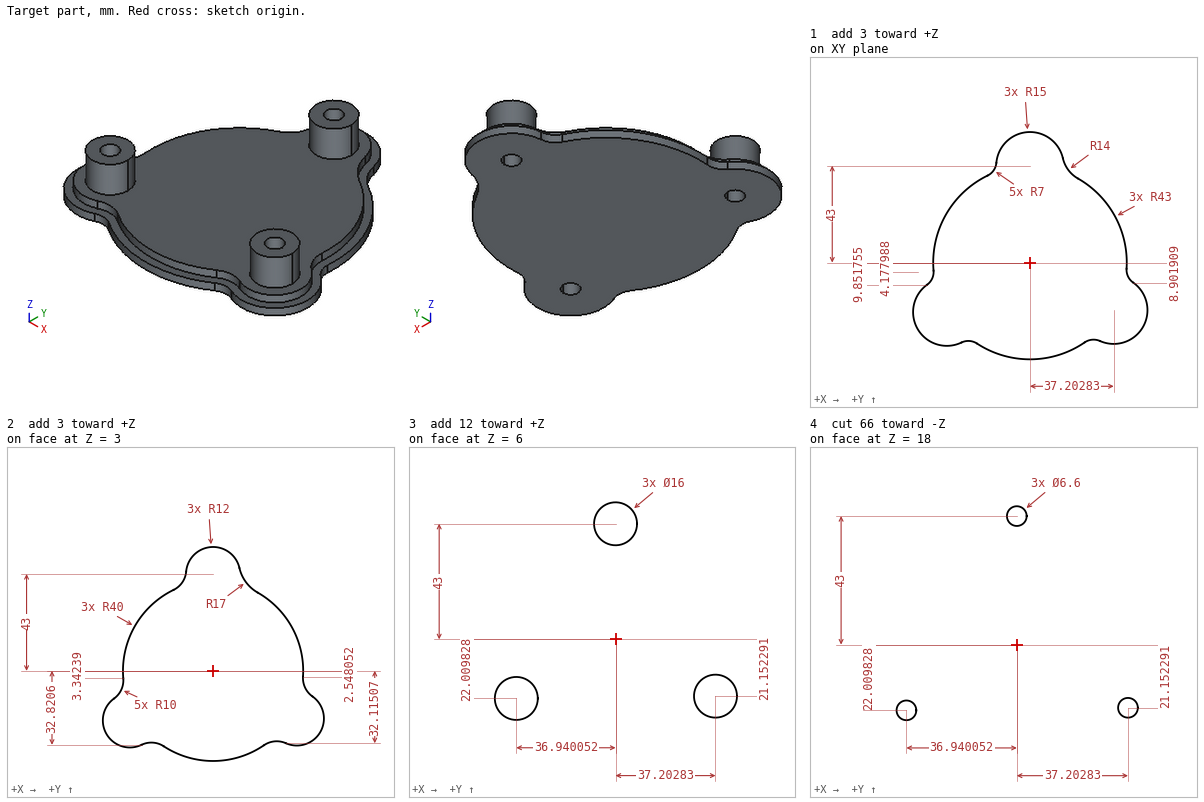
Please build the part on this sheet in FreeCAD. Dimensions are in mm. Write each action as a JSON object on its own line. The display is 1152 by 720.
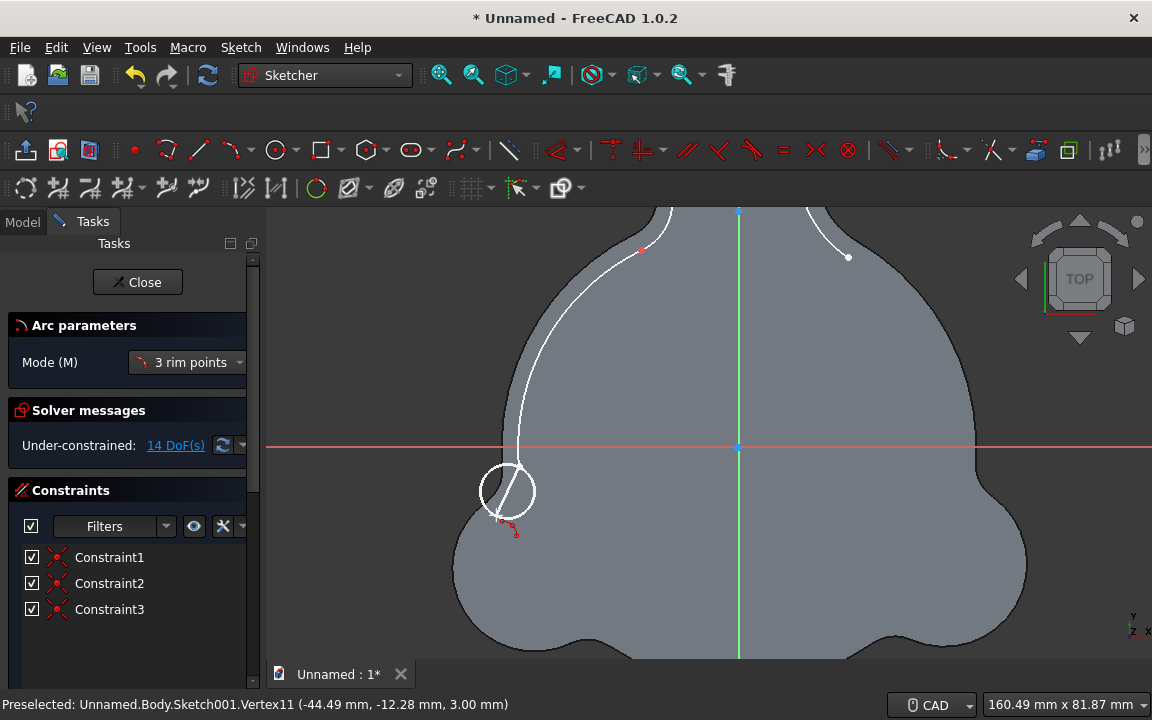
{"action": "scroll", "coordinate": [514, 493], "scroll_direction": "up", "scroll_amount": 4}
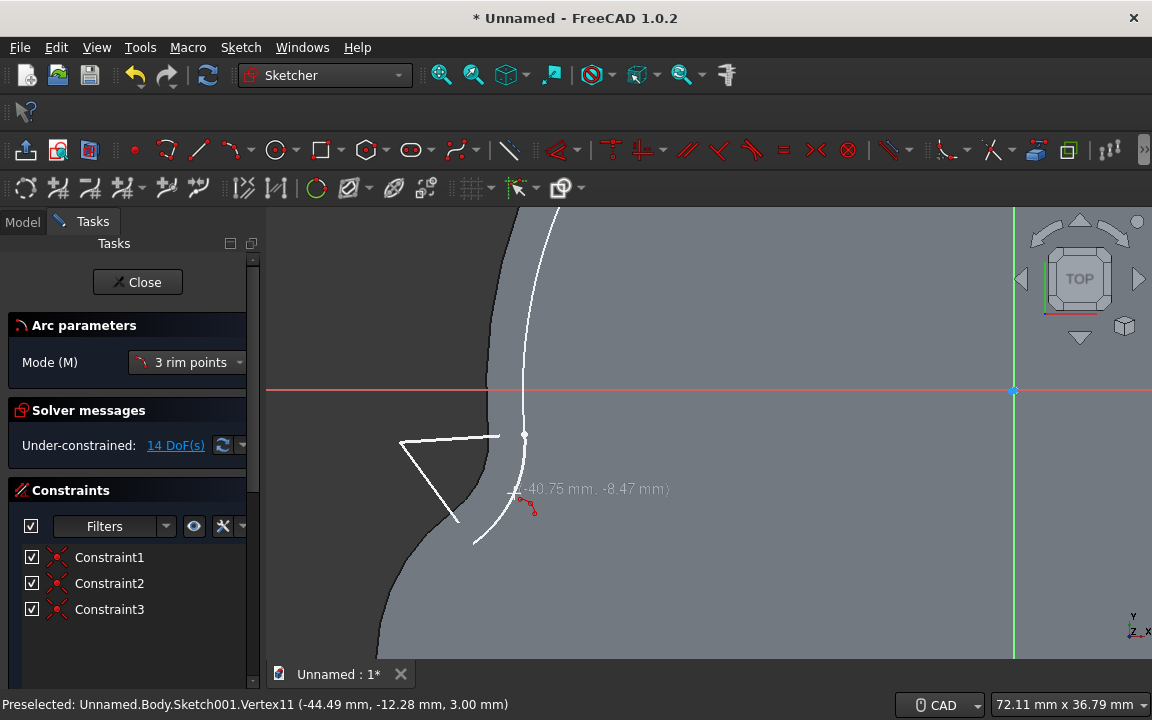
{"action": "left_click", "coordinate": [514, 493]}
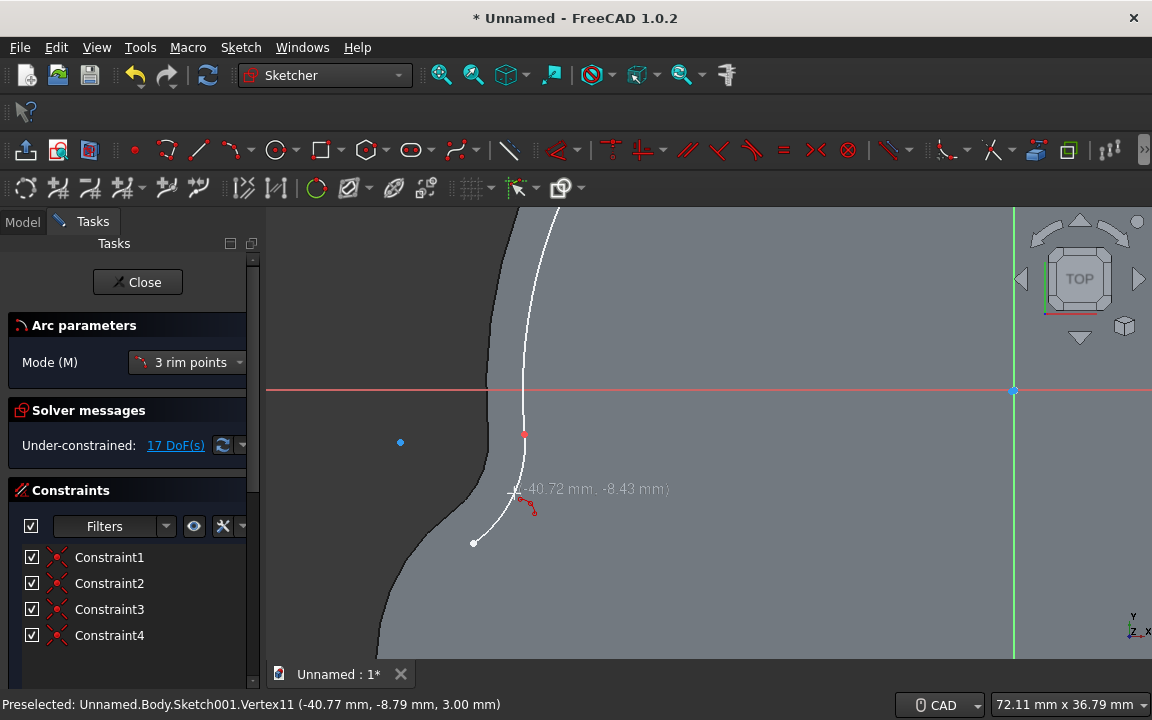
{"action": "scroll", "coordinate": [517, 477], "scroll_direction": "down", "scroll_amount": 7}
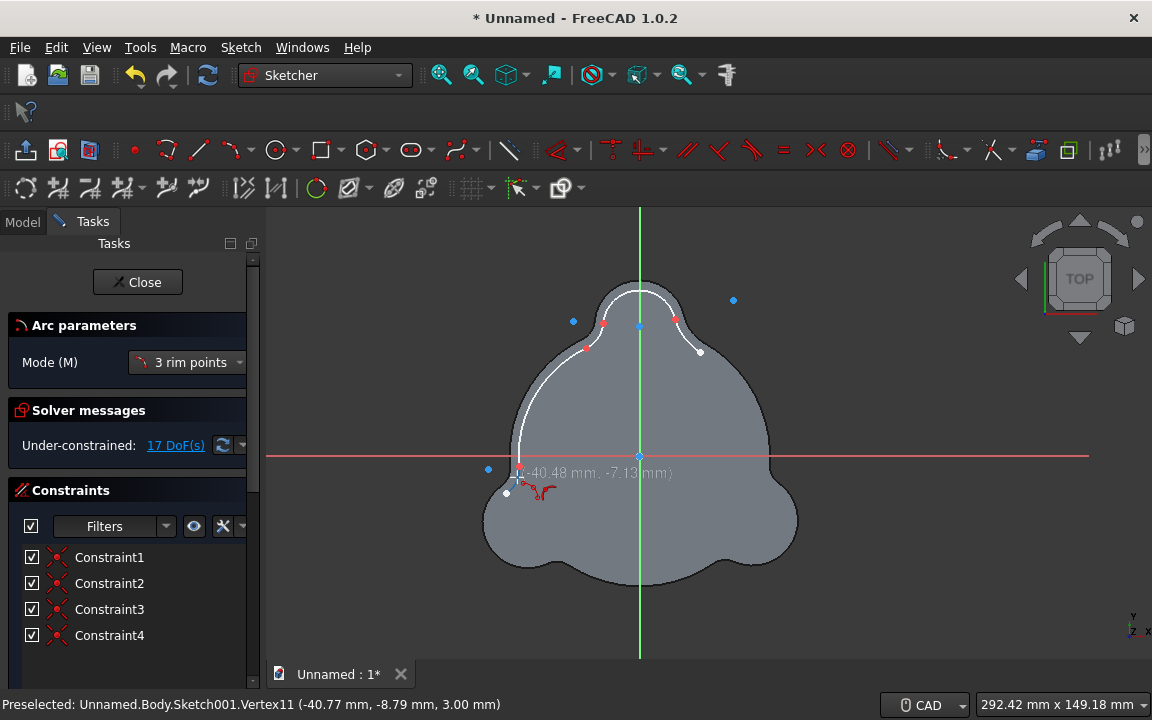
{"action": "left_click", "coordinate": [507, 494]}
{"action": "left_click", "coordinate": [544, 556]}
{"action": "left_click", "coordinate": [497, 541]}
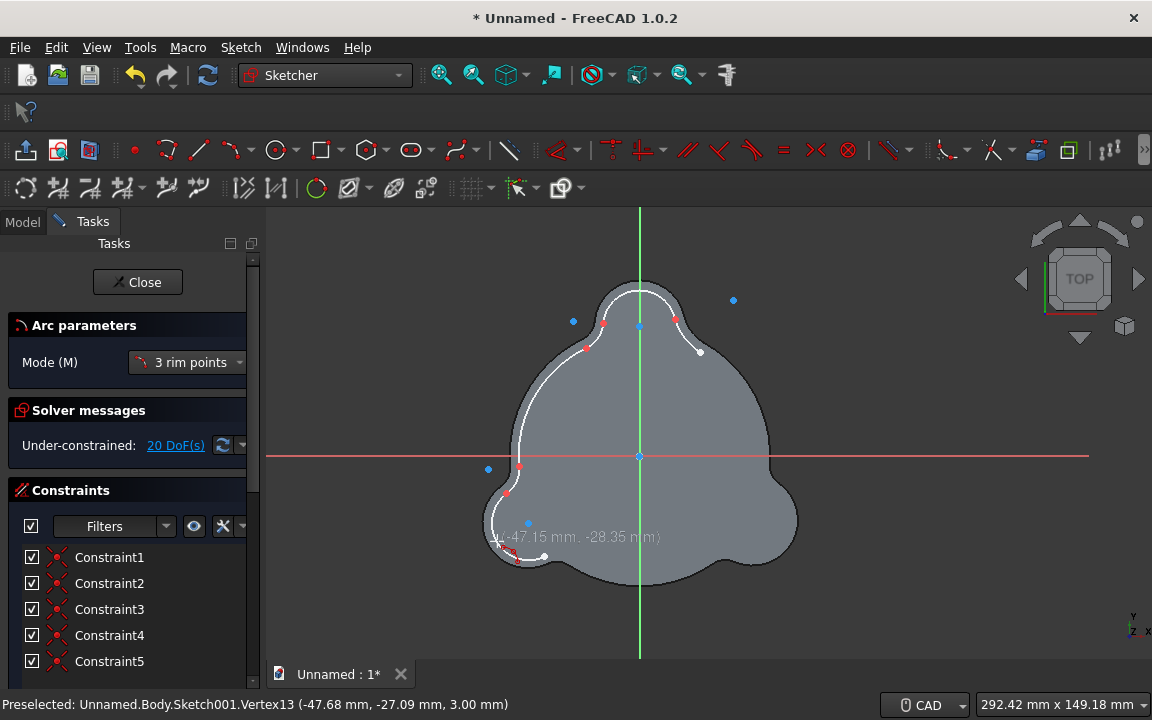
{"action": "left_click", "coordinate": [544, 557]}
{"action": "left_click", "coordinate": [573, 557]}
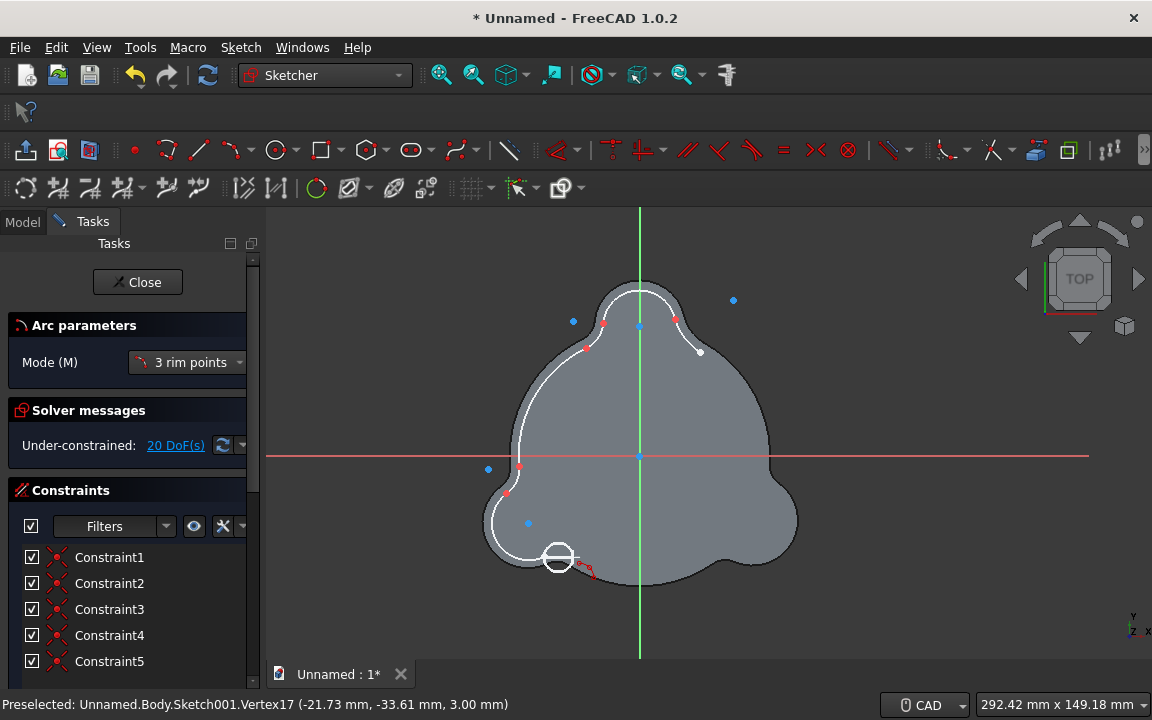
{"action": "scroll", "coordinate": [559, 553], "scroll_direction": "up", "scroll_amount": 7}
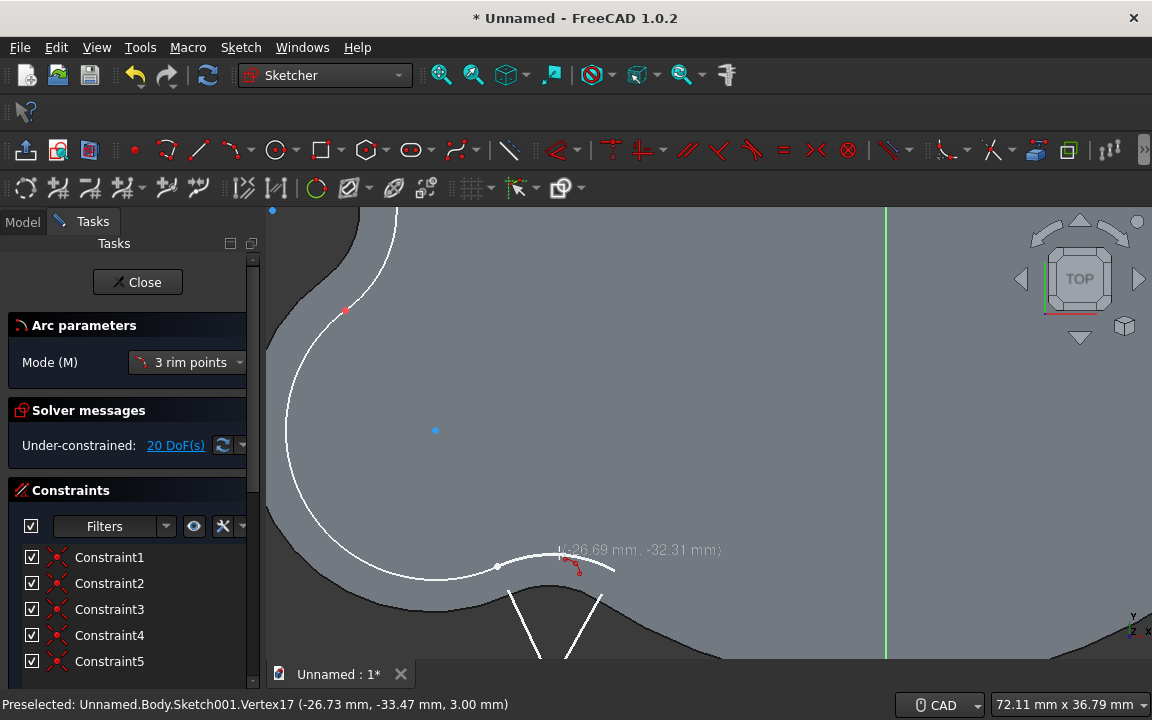
{"action": "left_click", "coordinate": [557, 549]}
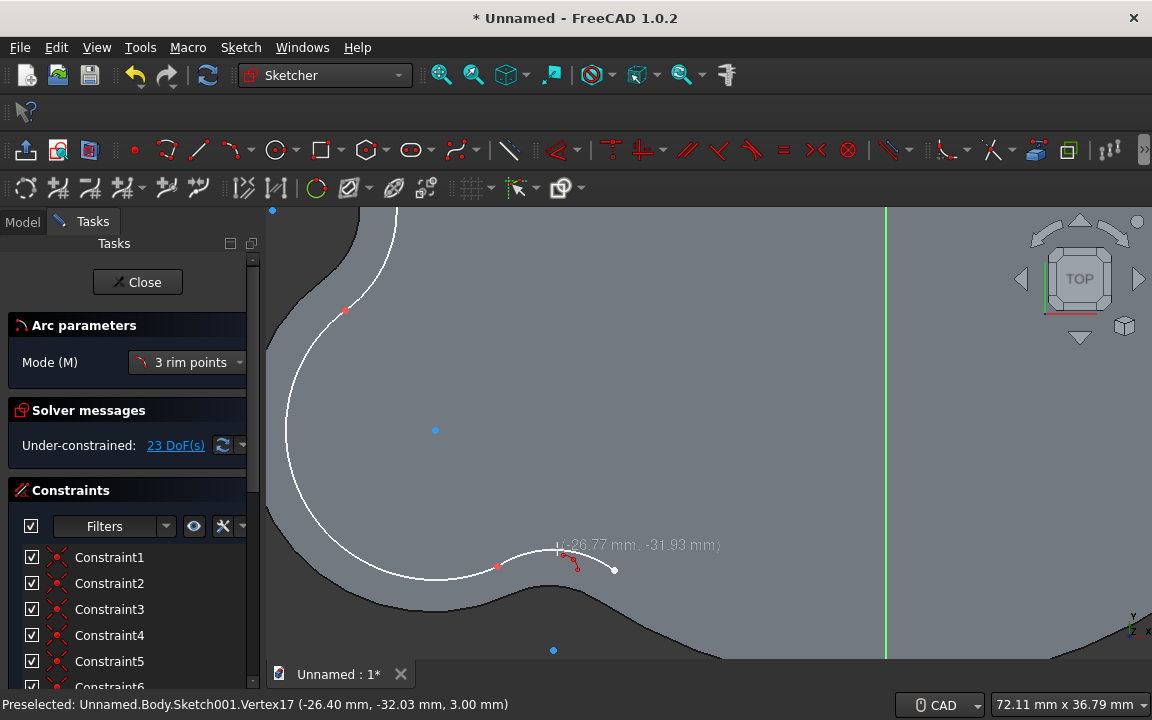
{"action": "scroll", "coordinate": [559, 553], "scroll_direction": "down", "scroll_amount": 7}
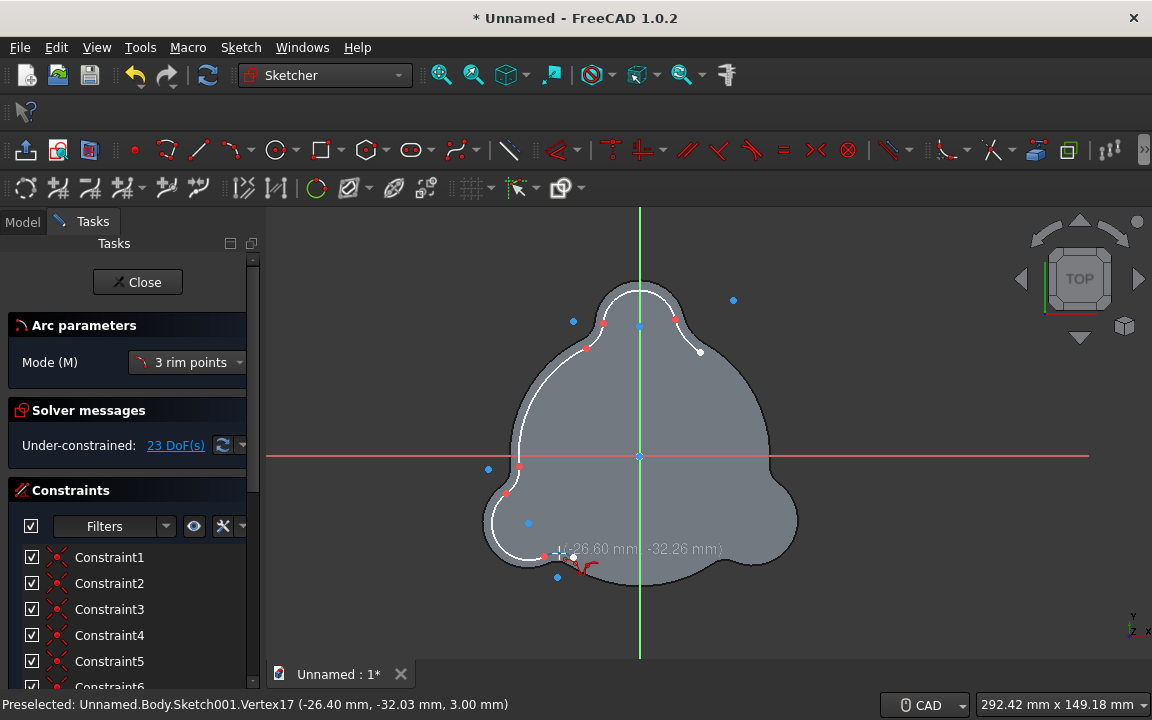
{"action": "left_click", "coordinate": [573, 558]}
{"action": "left_click", "coordinate": [708, 556]}
{"action": "left_click", "coordinate": [655, 576]}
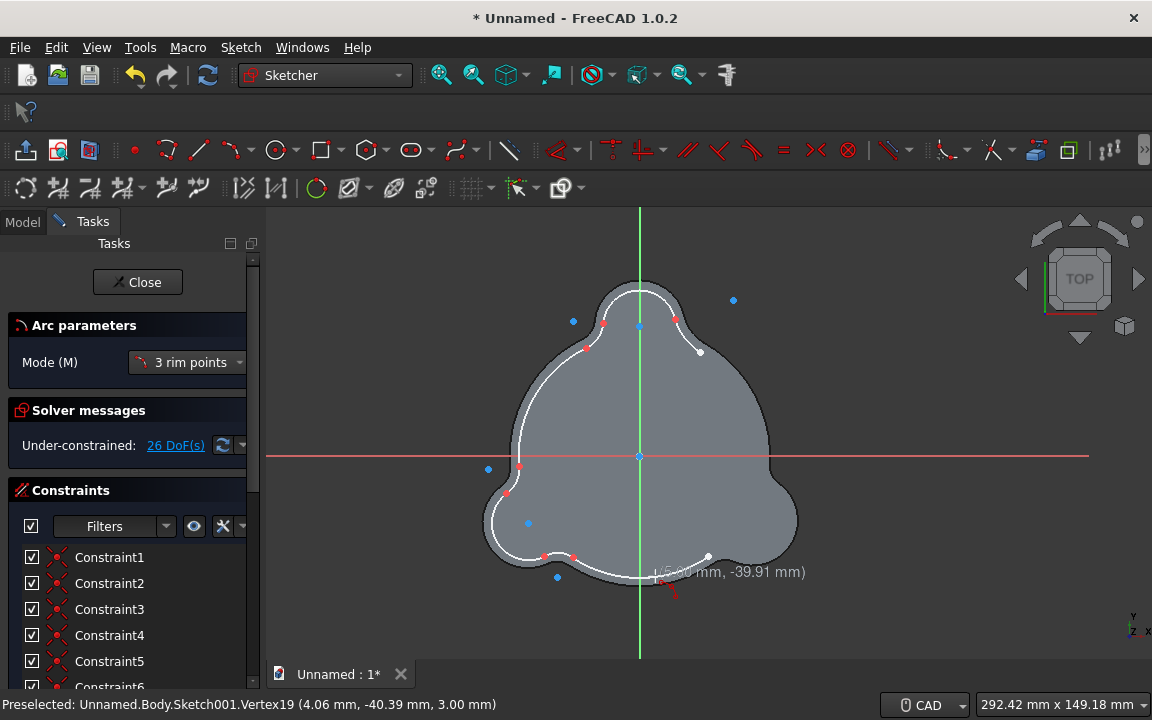
{"action": "left_click", "coordinate": [708, 557]}
{"action": "left_click", "coordinate": [738, 553]}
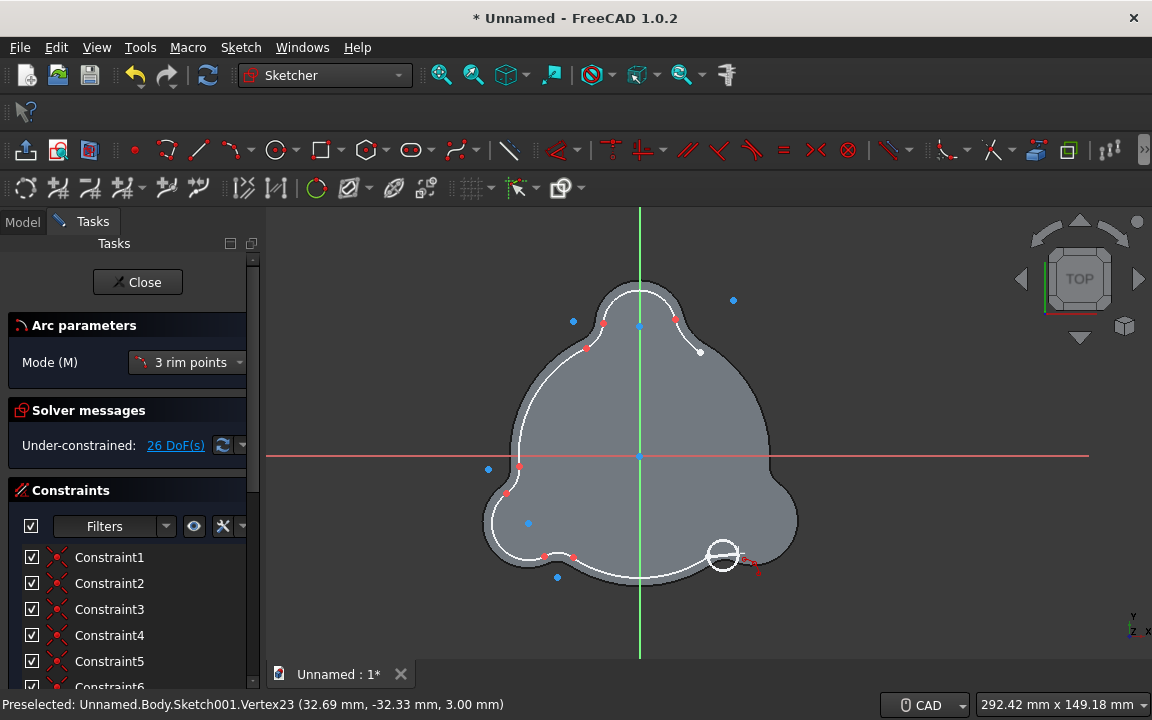
{"action": "scroll", "coordinate": [723, 551], "scroll_direction": "up", "scroll_amount": 8}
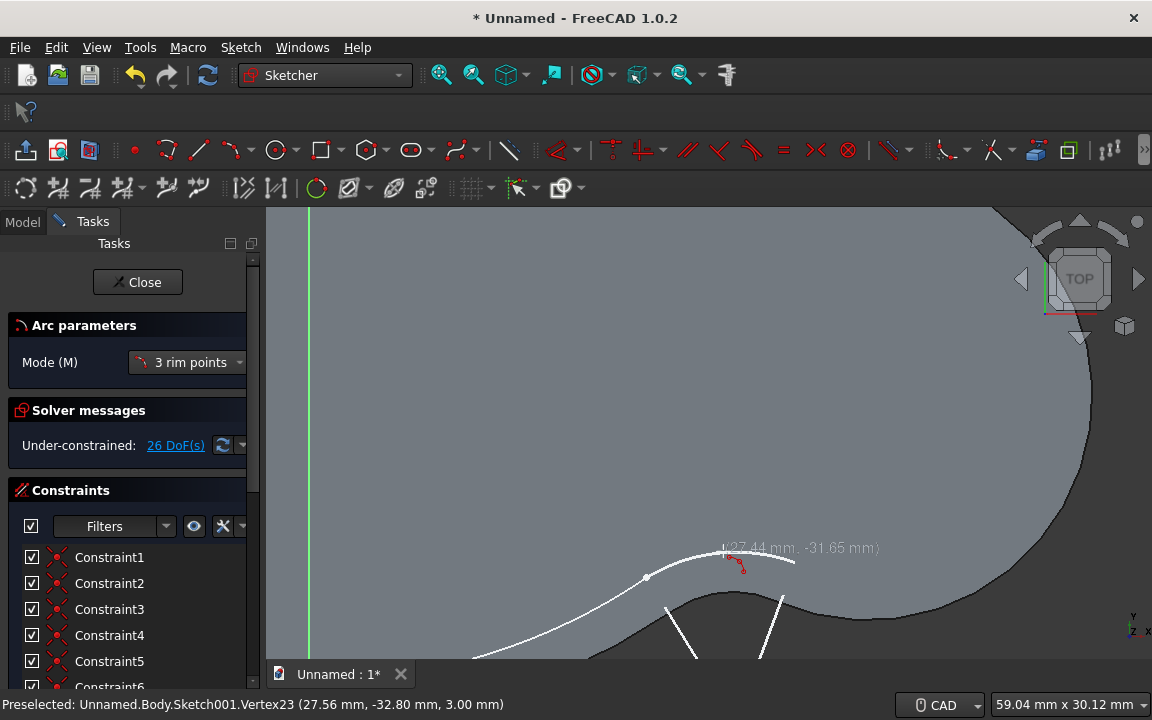
{"action": "left_click", "coordinate": [720, 547]}